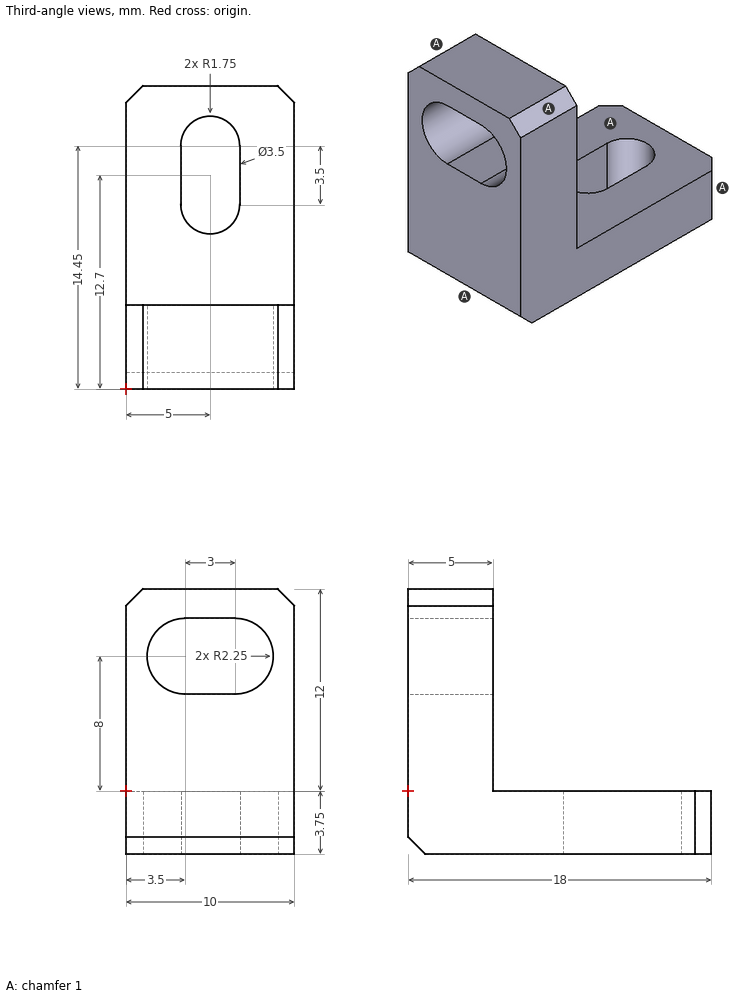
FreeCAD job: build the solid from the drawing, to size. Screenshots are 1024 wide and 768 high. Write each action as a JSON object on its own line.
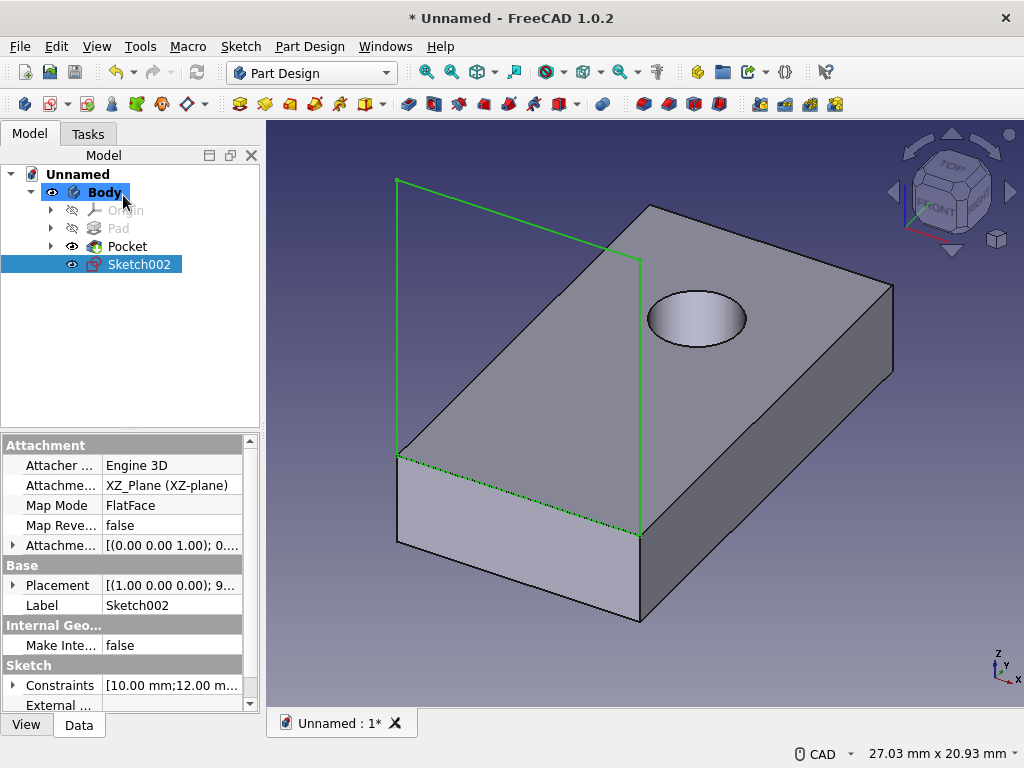
{"action": "left_click", "coordinate": [240, 104]}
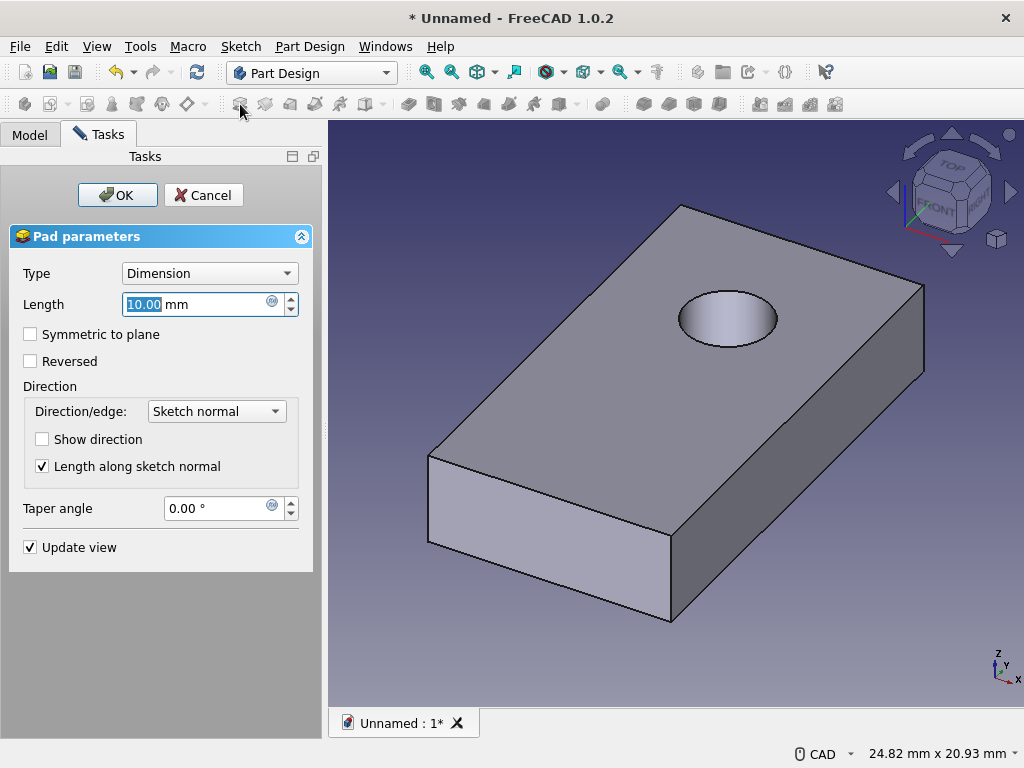
{"action": "type", "text": "5"}
{"action": "key", "text": "Tab"}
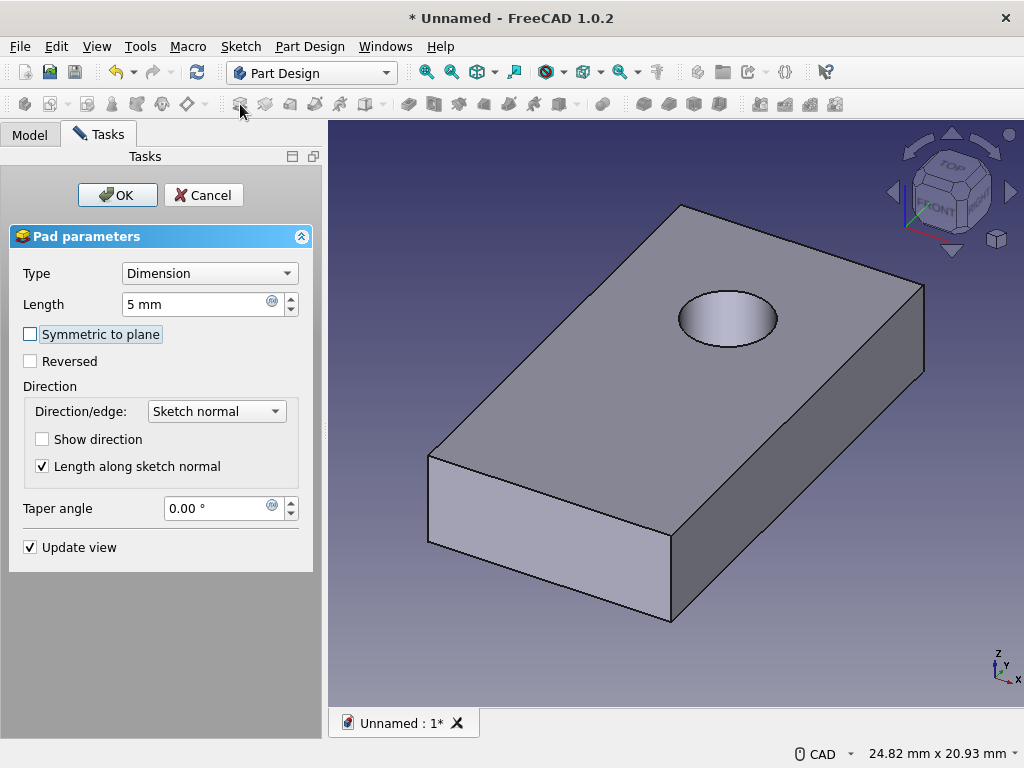
{"action": "left_click", "coordinate": [31, 361]}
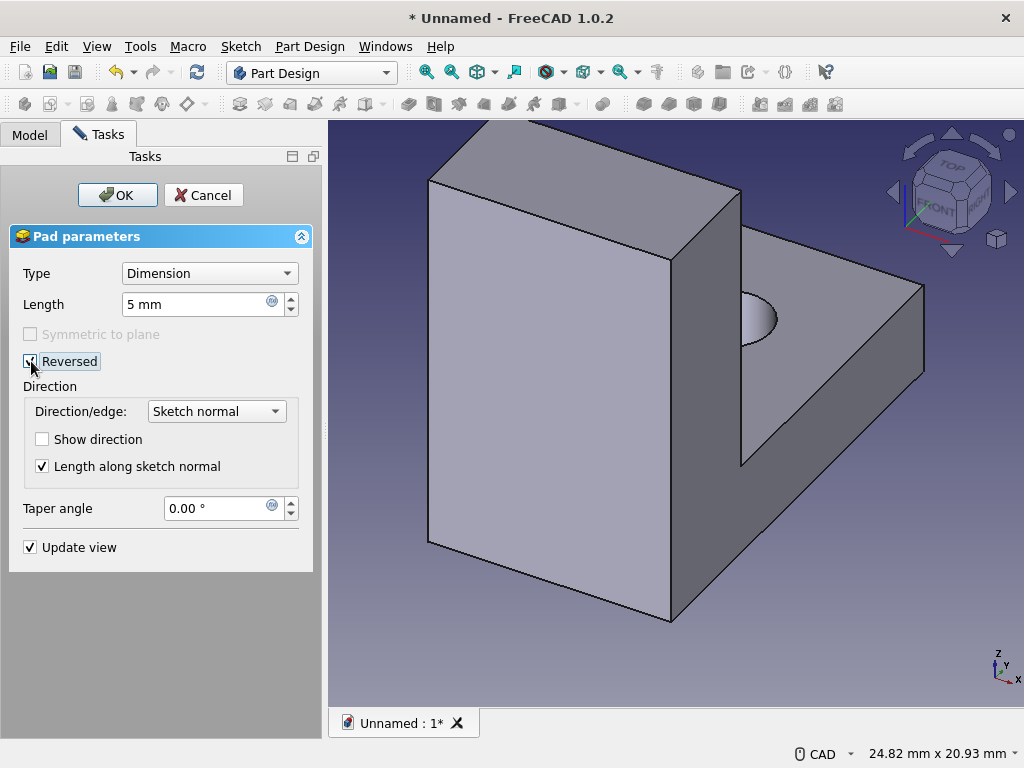
{"action": "left_click", "coordinate": [118, 195]}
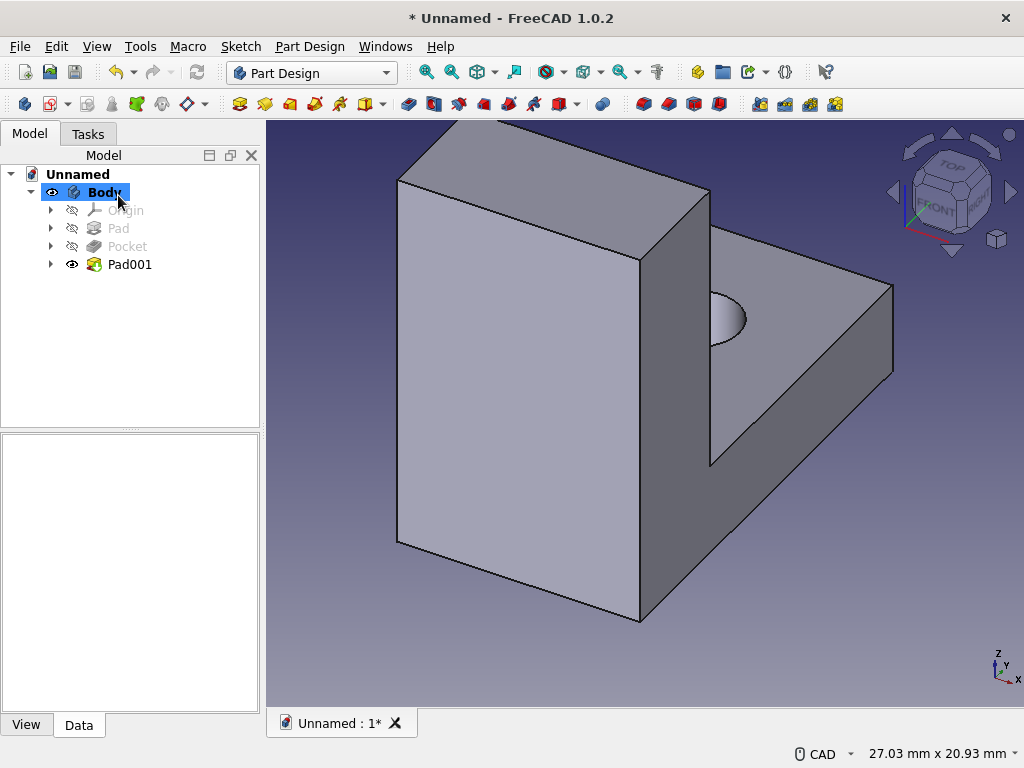
{"action": "key", "text": "v f"}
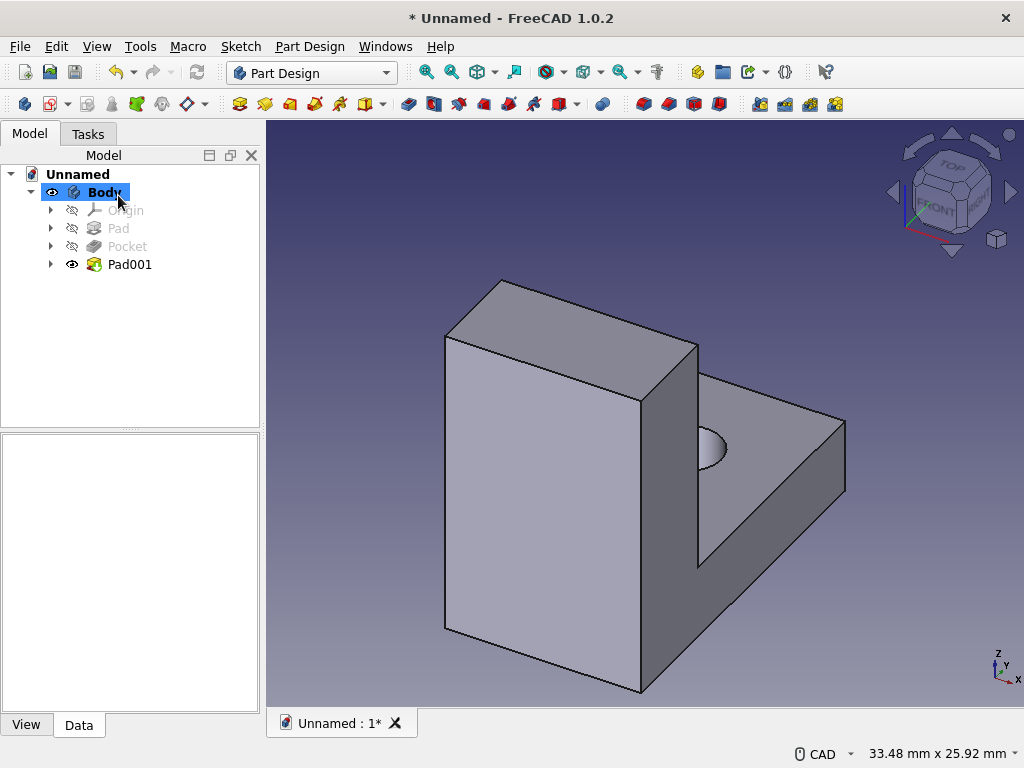
{"action": "key", "text": "4"}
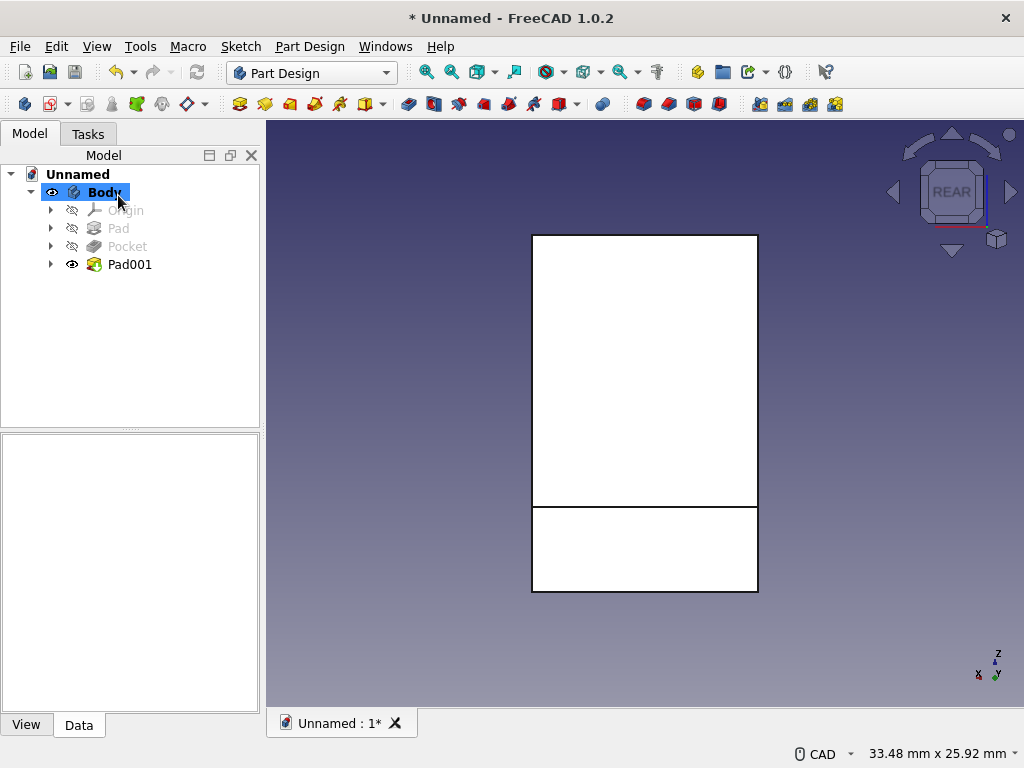
{"action": "left_click", "coordinate": [645, 370]}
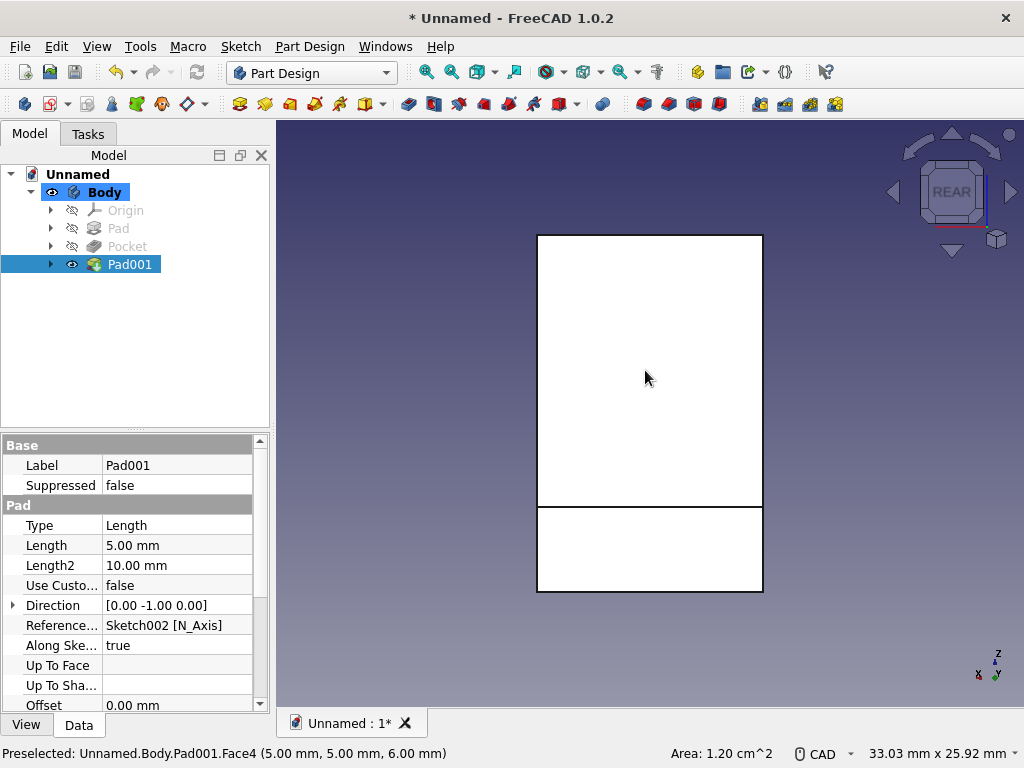
{"action": "left_click", "coordinate": [50, 104]}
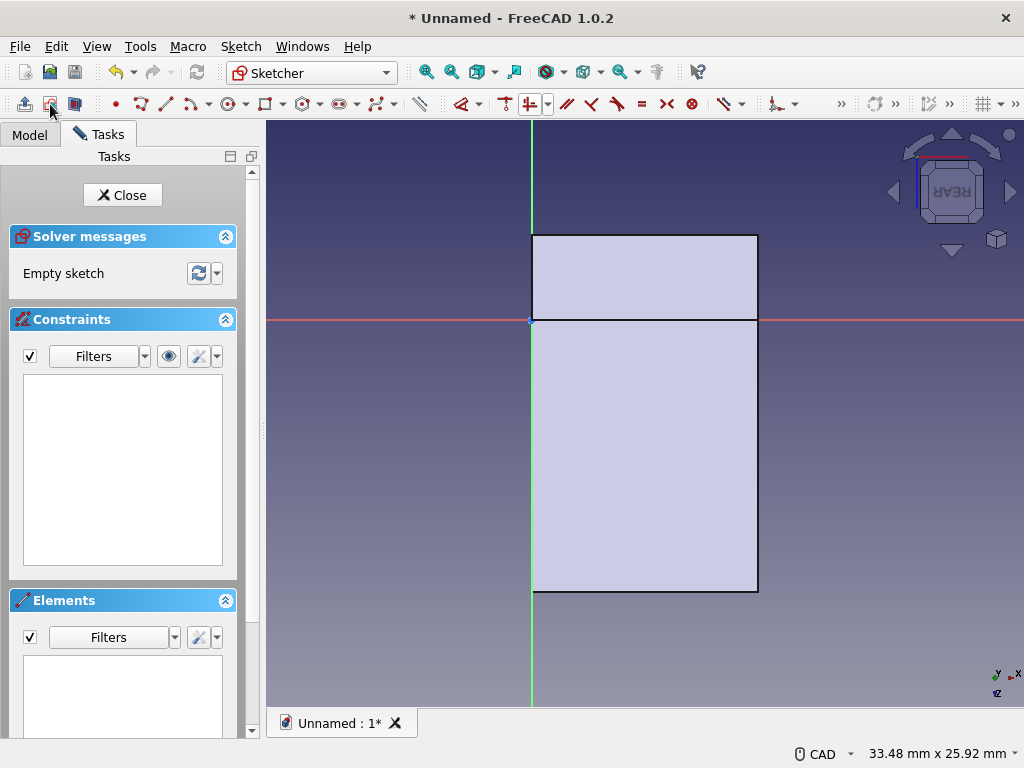
{"action": "scroll", "coordinate": [741, 482], "scroll_direction": "up", "scroll_amount": 2}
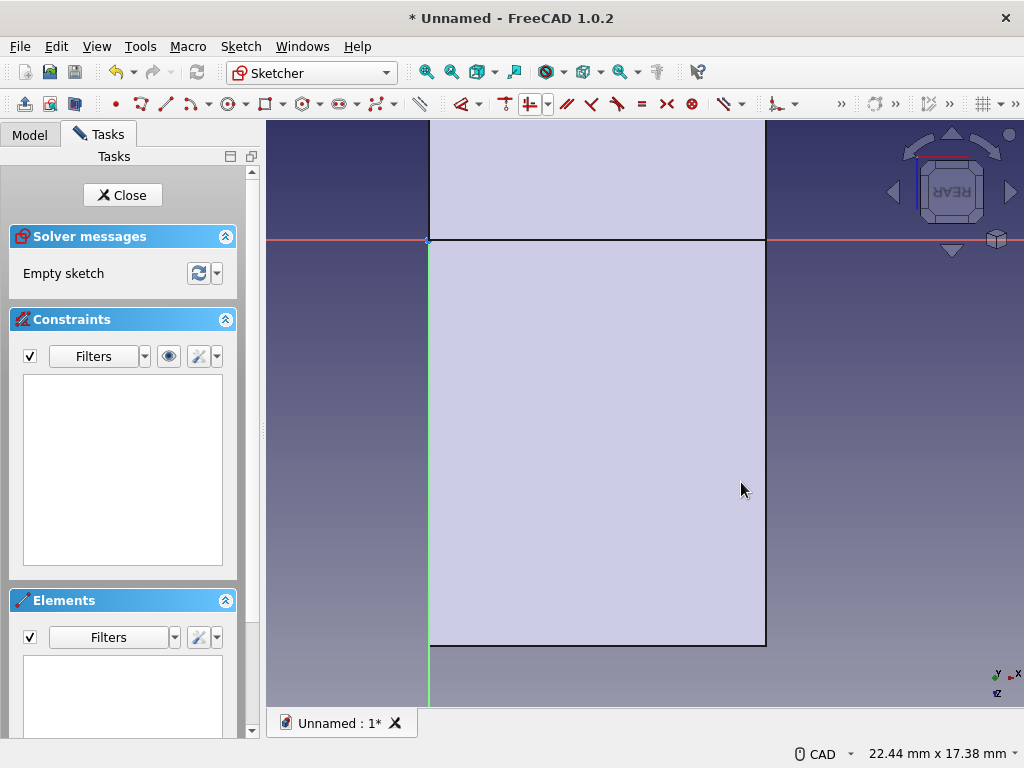
{"action": "left_click", "coordinate": [338, 104]}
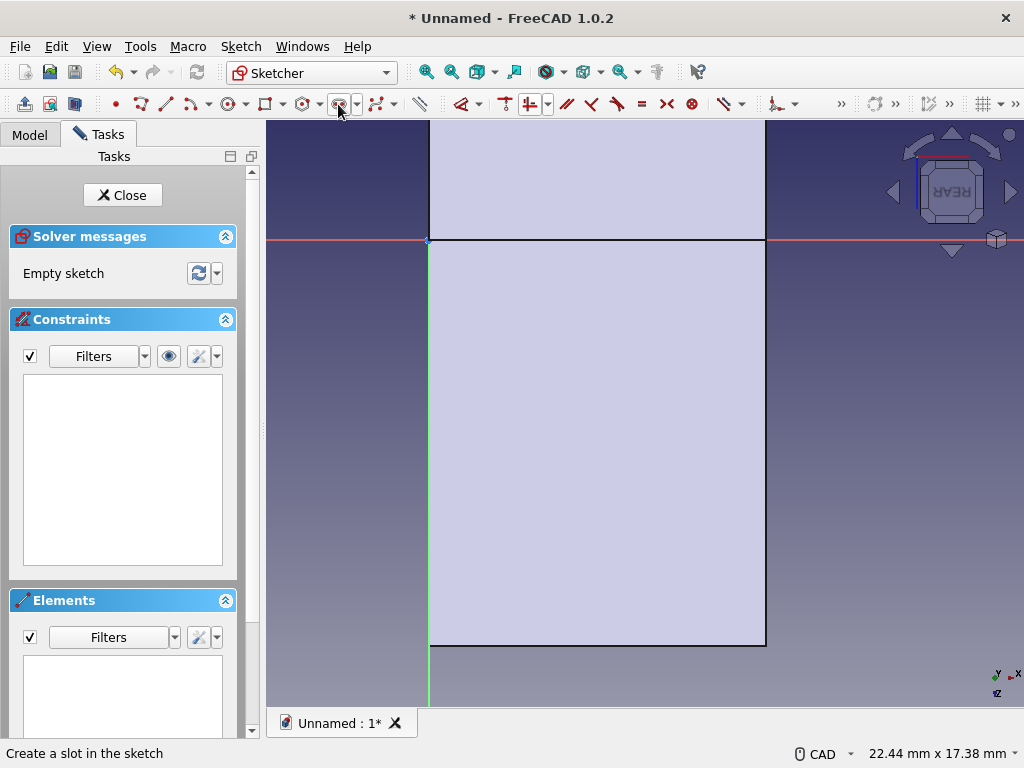
{"action": "left_click", "coordinate": [547, 510]}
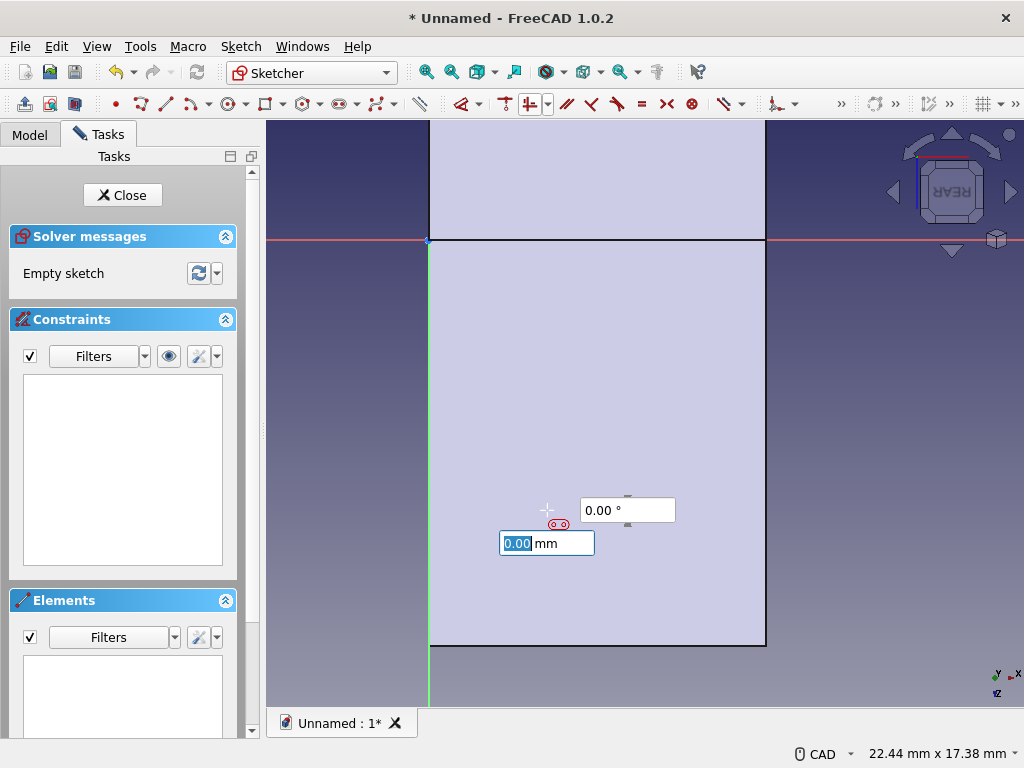
{"action": "left_click", "coordinate": [648, 510]}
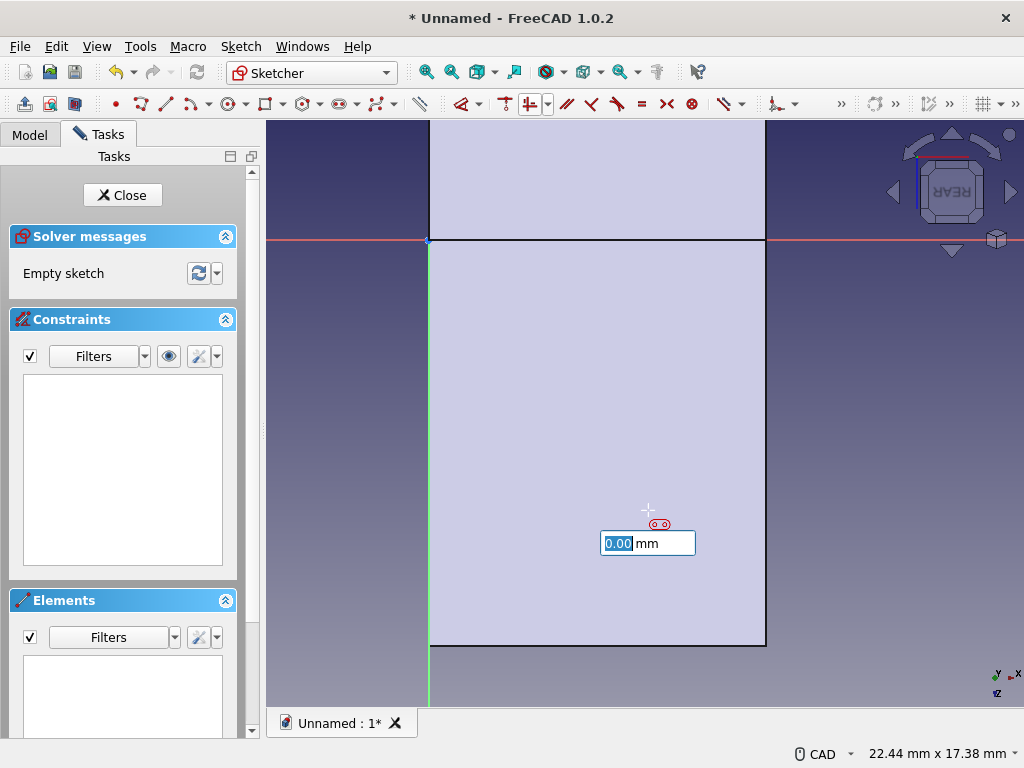
{"action": "left_click", "coordinate": [597, 586]}
{"action": "key", "text": "Escape"}